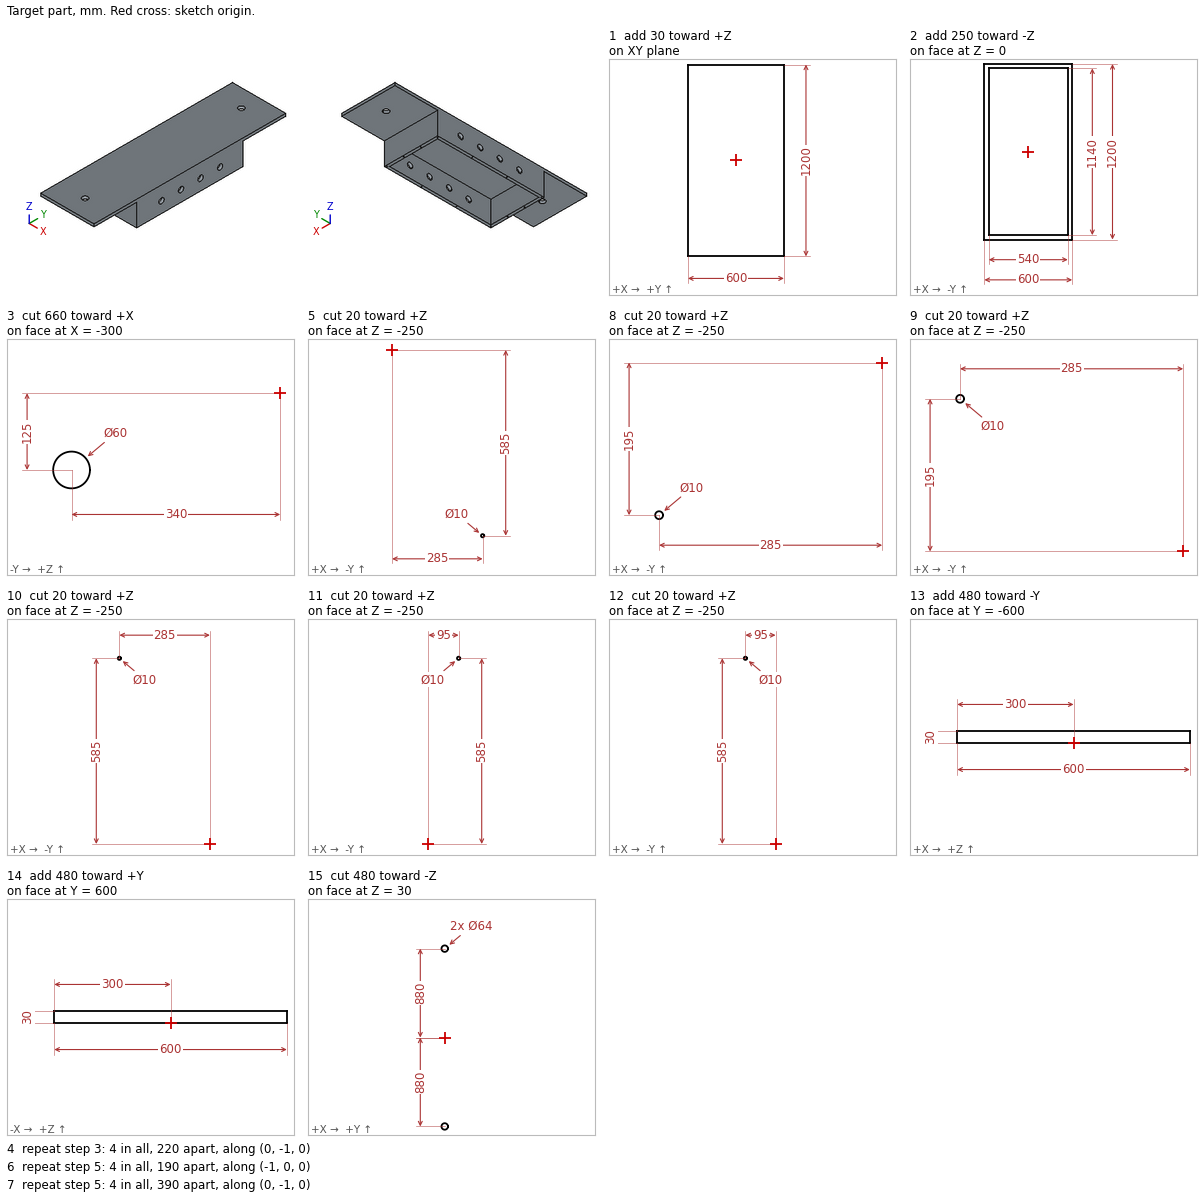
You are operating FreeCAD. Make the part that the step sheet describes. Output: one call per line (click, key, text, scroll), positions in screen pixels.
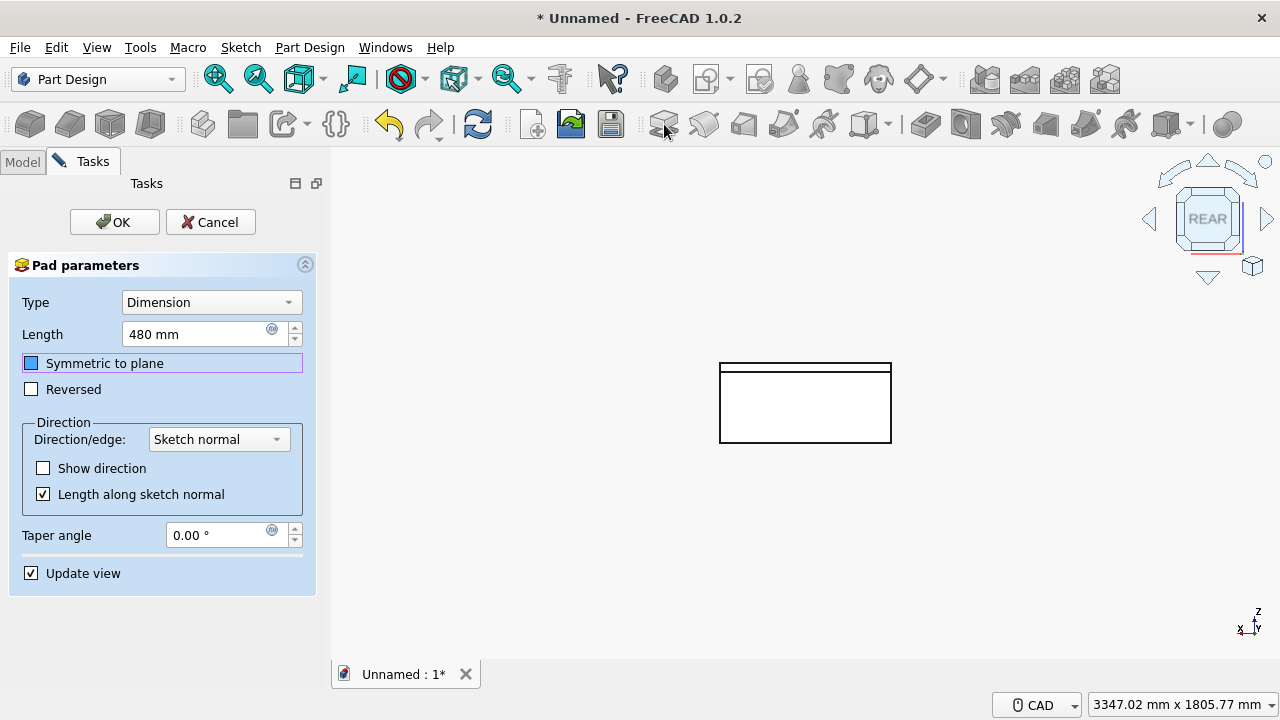
click(115, 222)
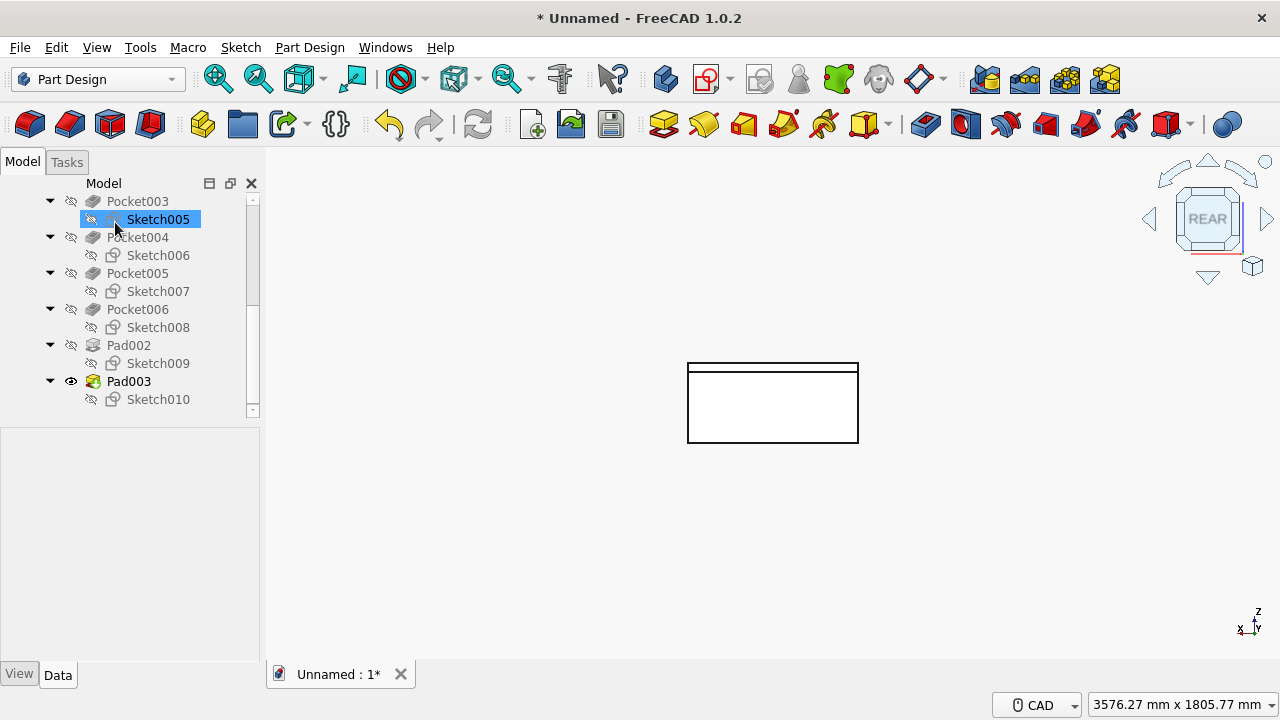
click(220, 80)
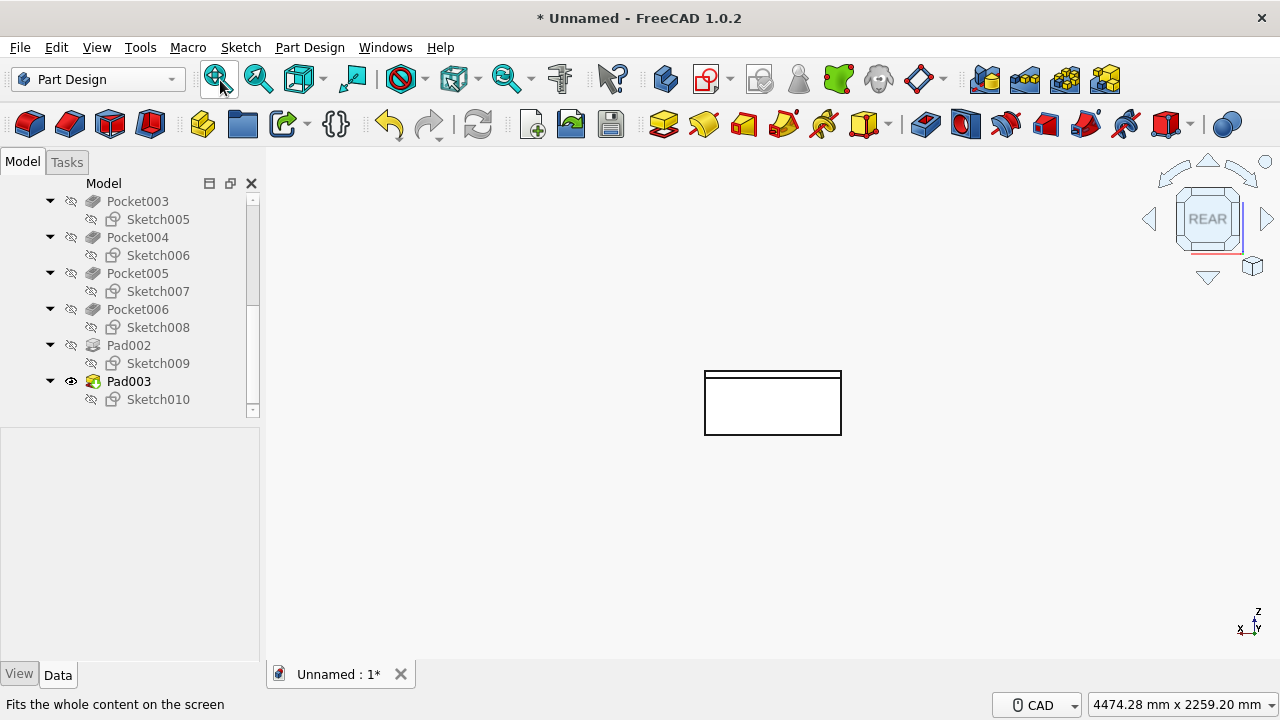
key(0)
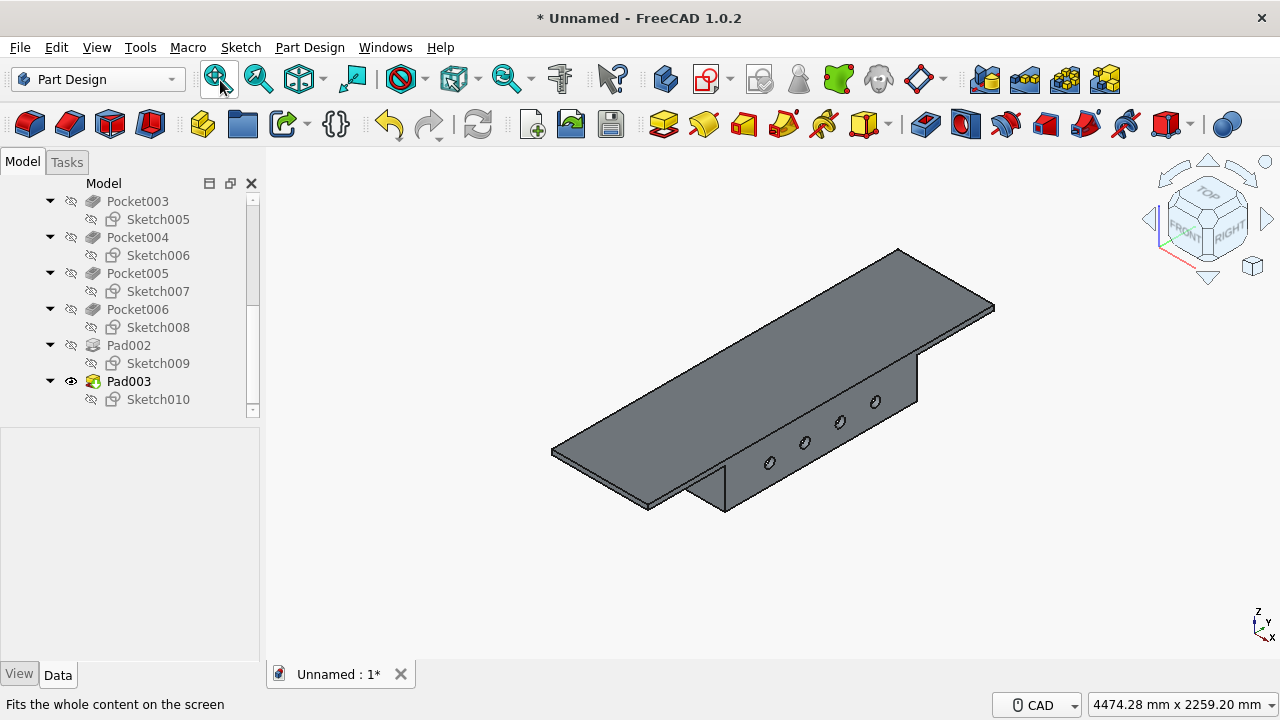
click(872, 319)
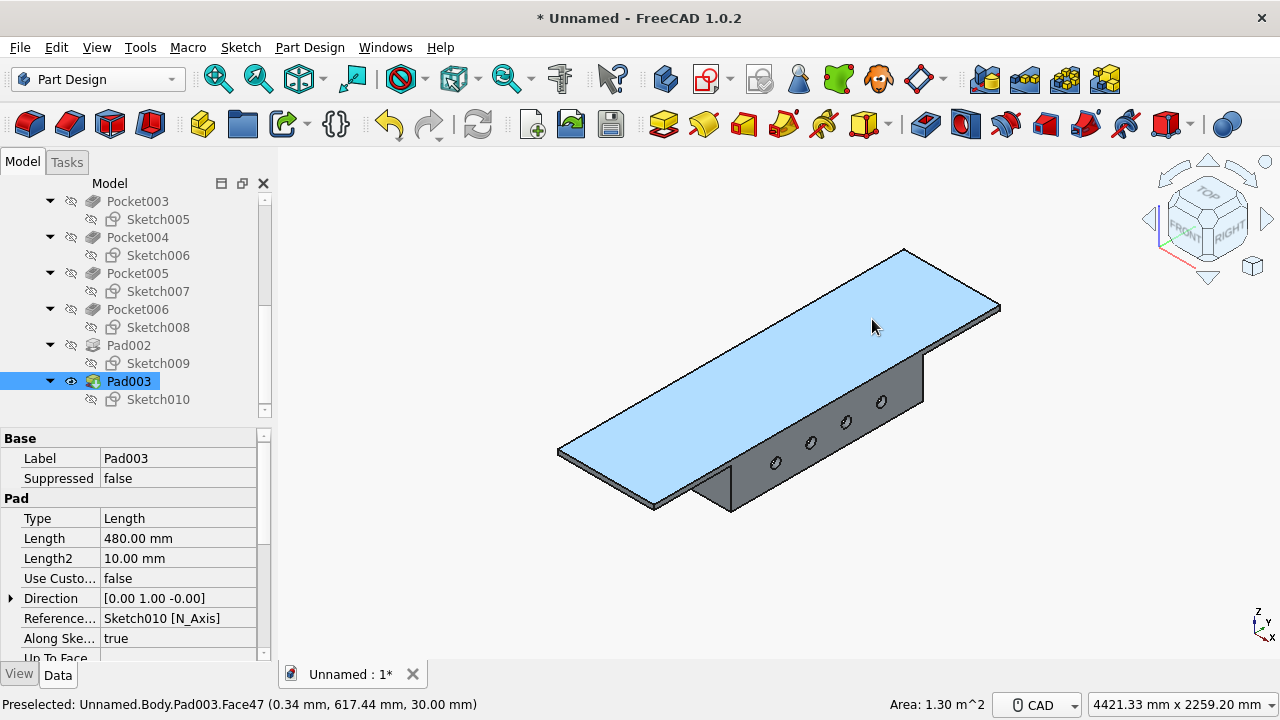
click(706, 80)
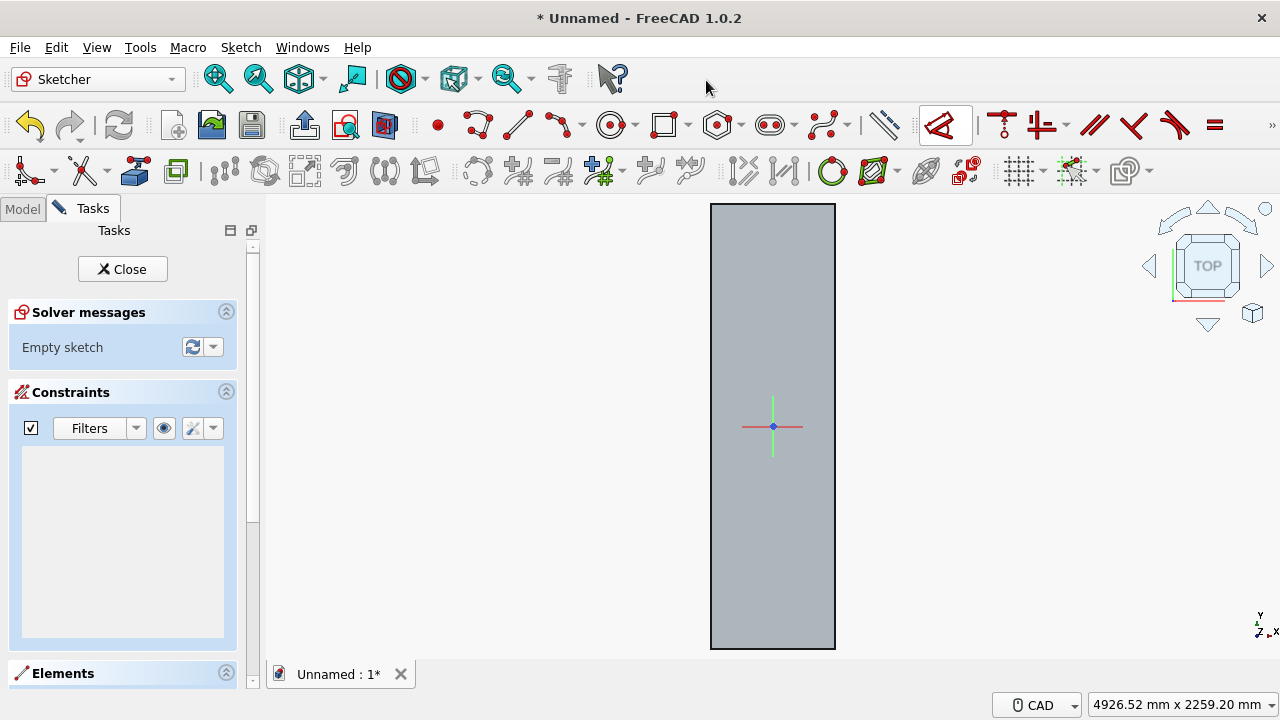
scroll(395, 426, down, 1)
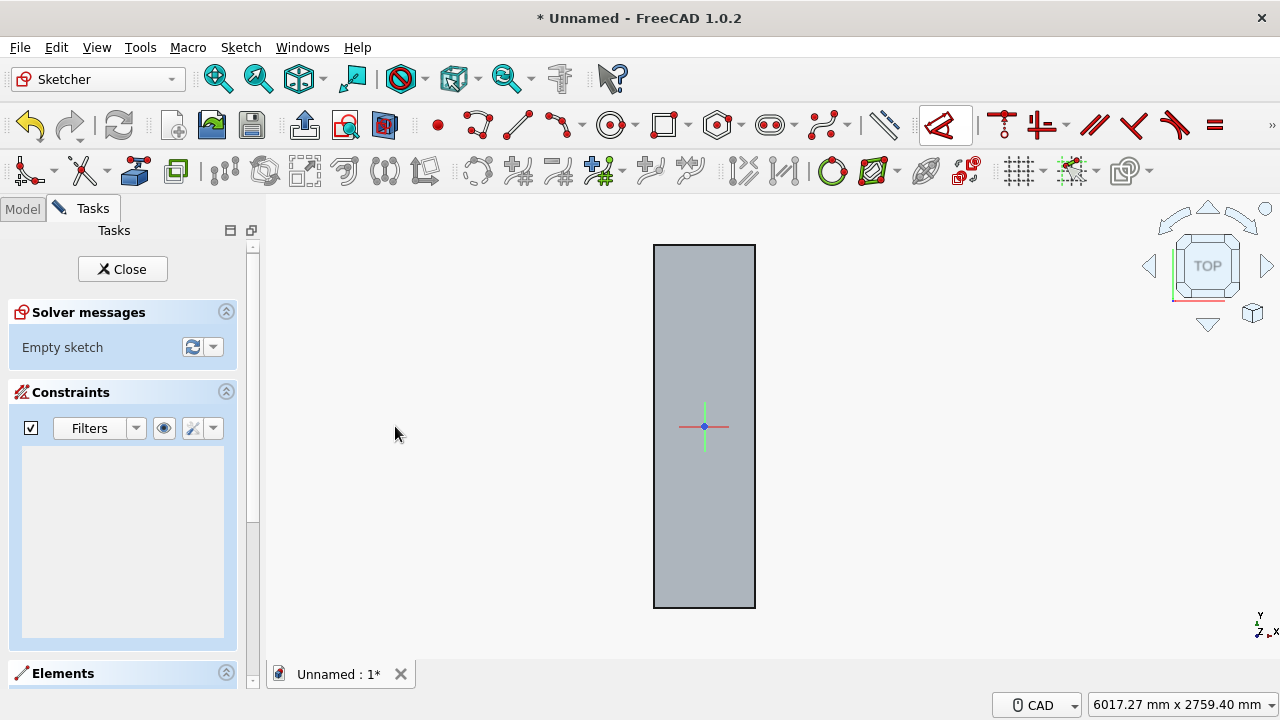
click(612, 126)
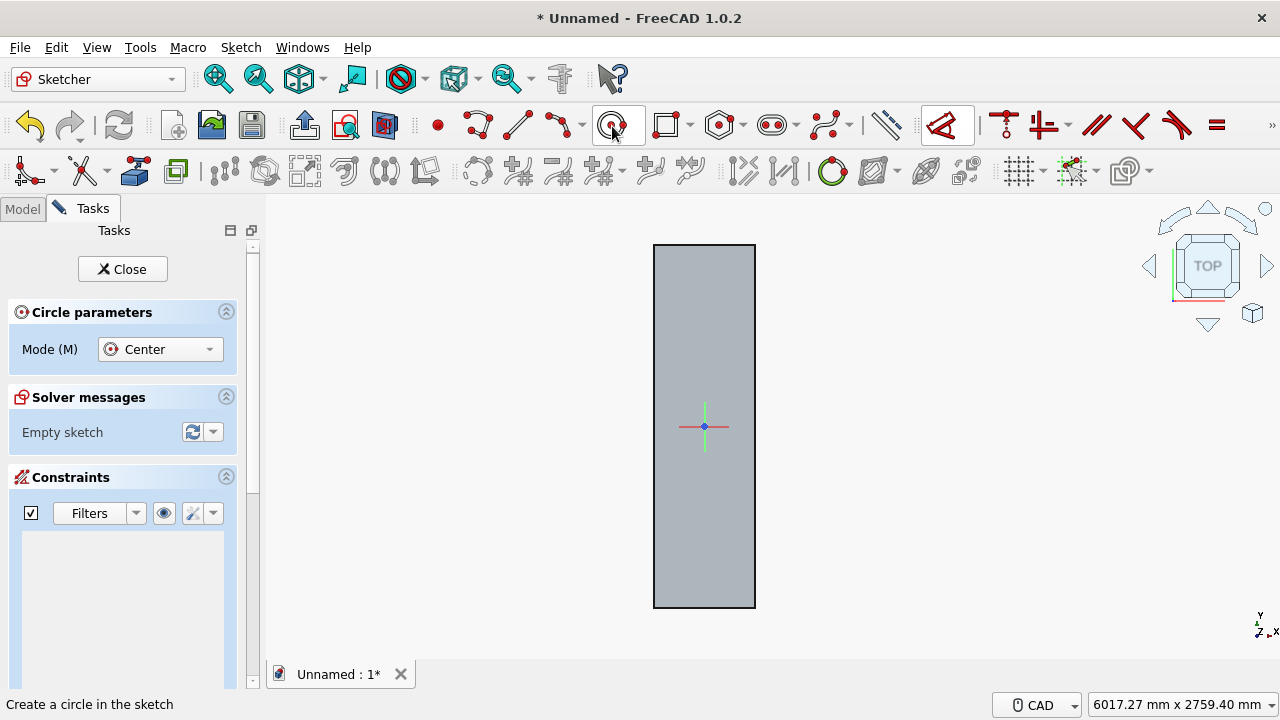
scroll(705, 278, up, 8)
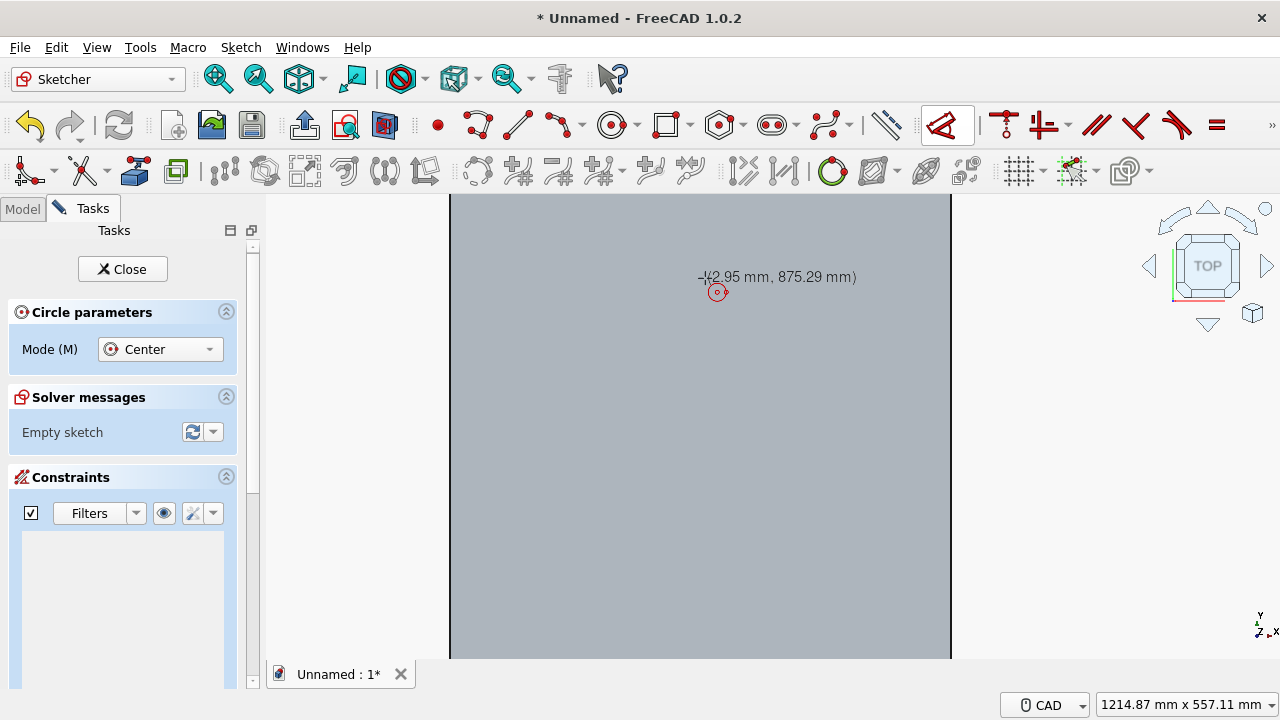
scroll(705, 278, down, 8)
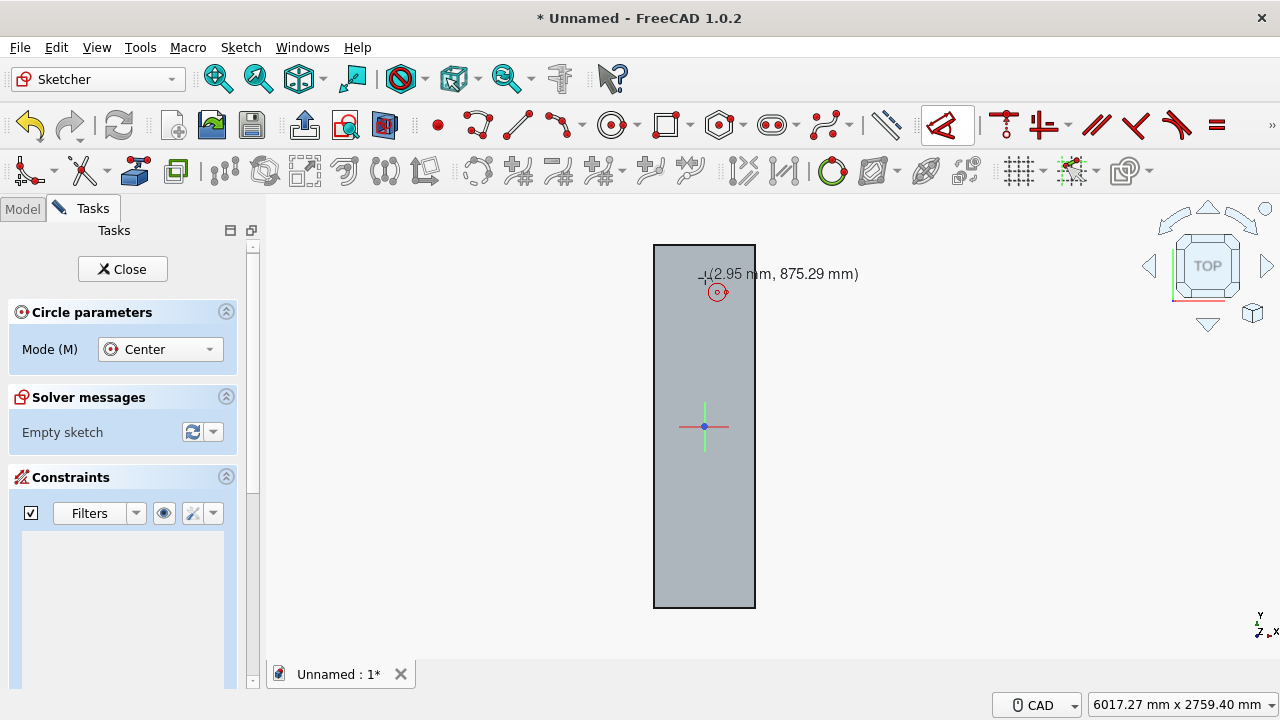
click(705, 278)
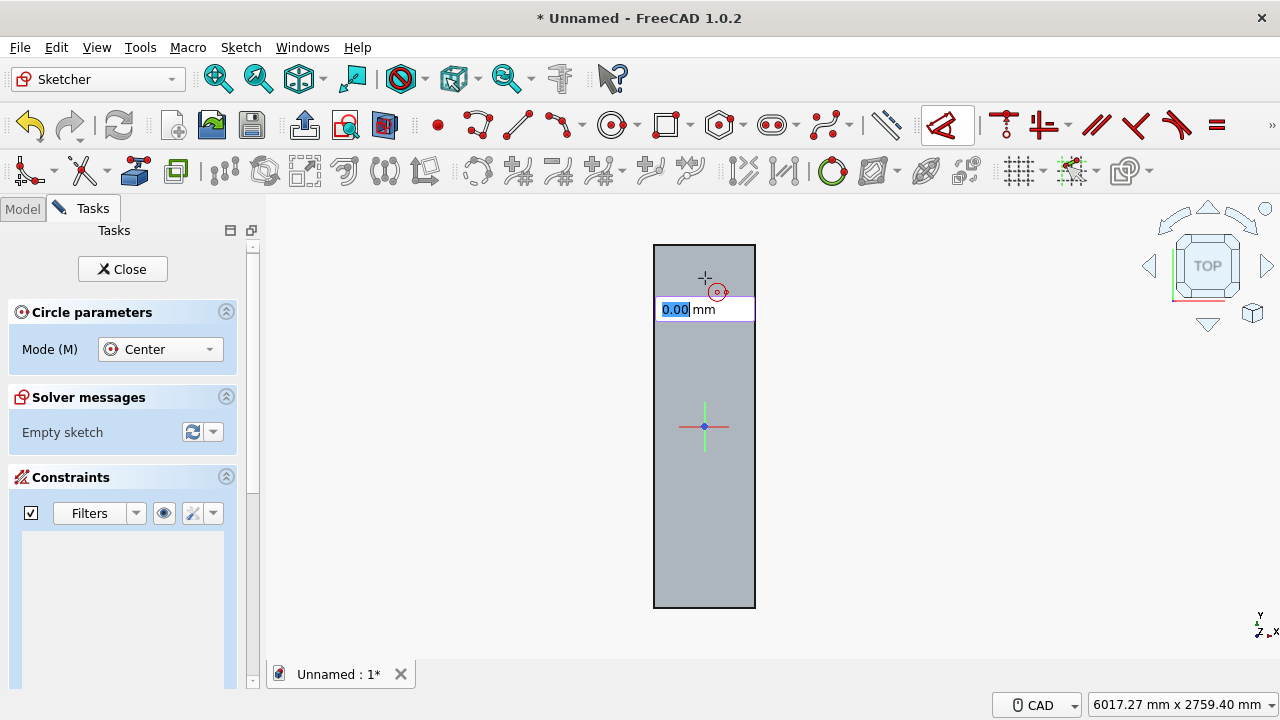
scroll(710, 276, up, 6)
move(708, 277)